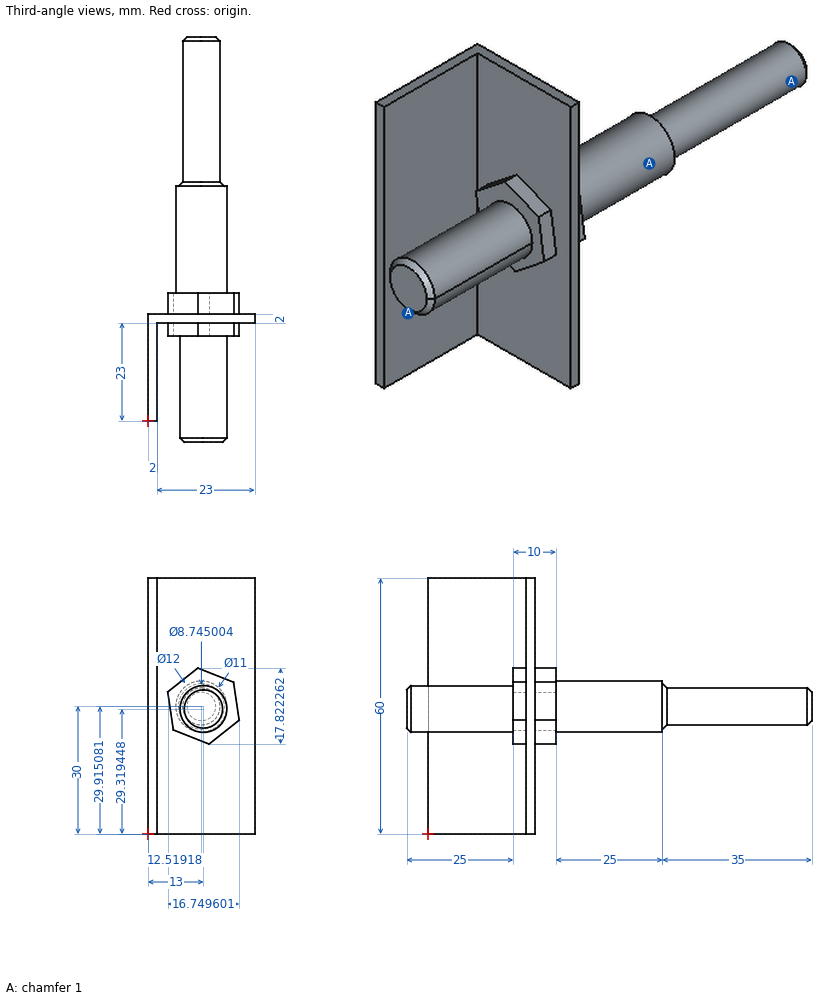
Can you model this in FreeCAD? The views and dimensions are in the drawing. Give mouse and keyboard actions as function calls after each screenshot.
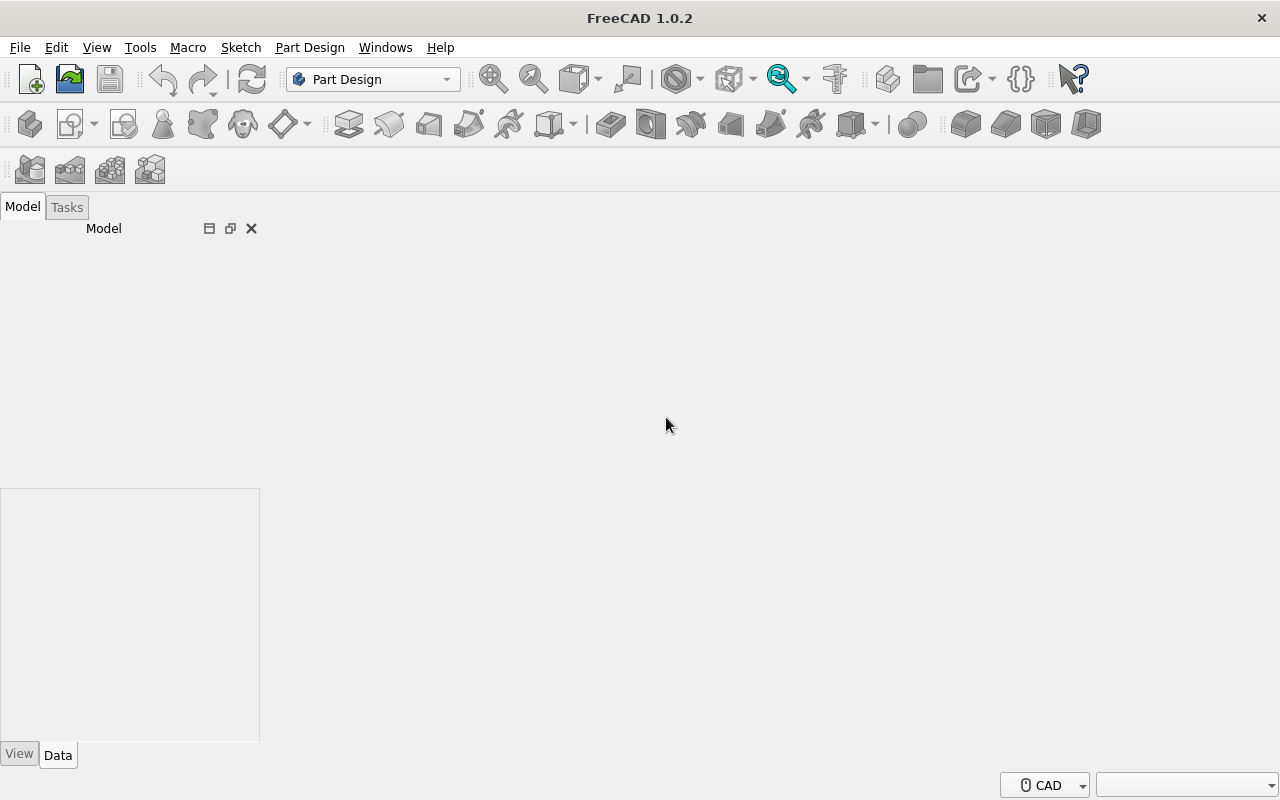
click(30, 80)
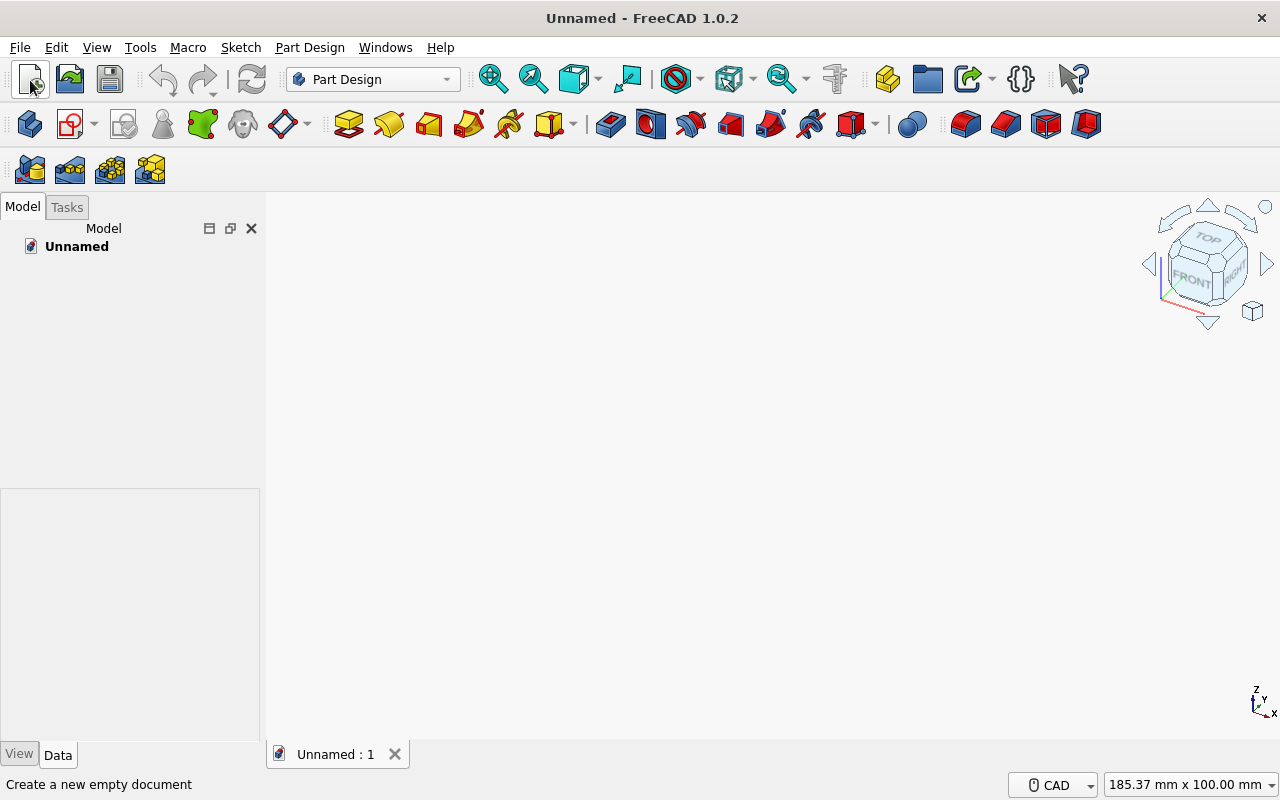
click(70, 124)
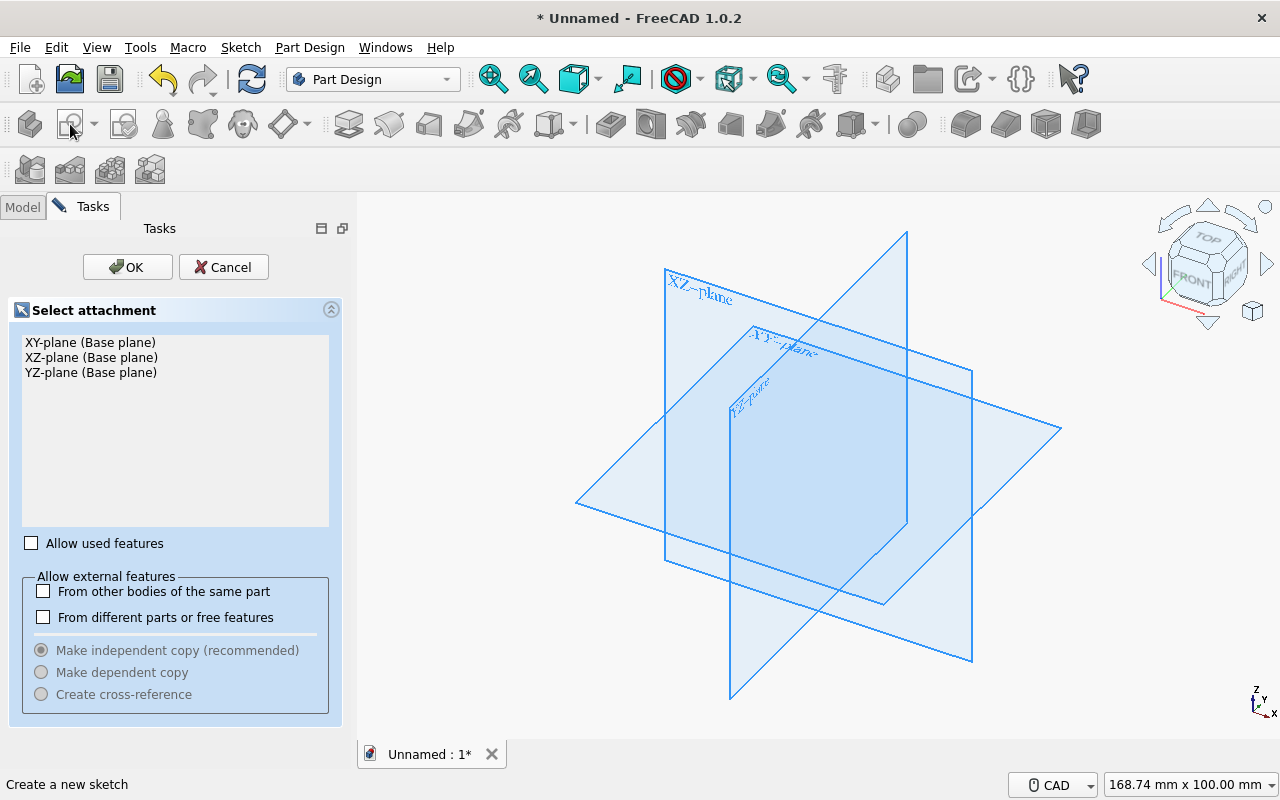
click(82, 342)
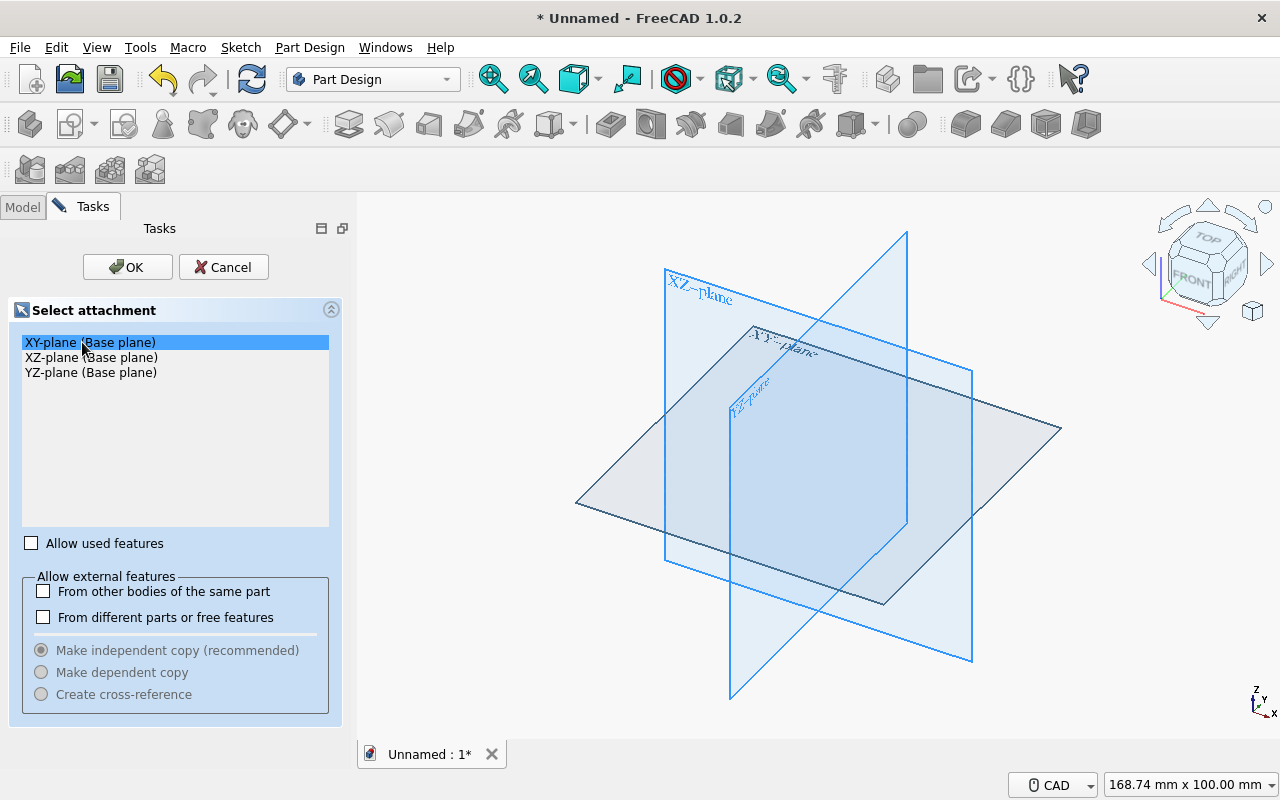
click(128, 267)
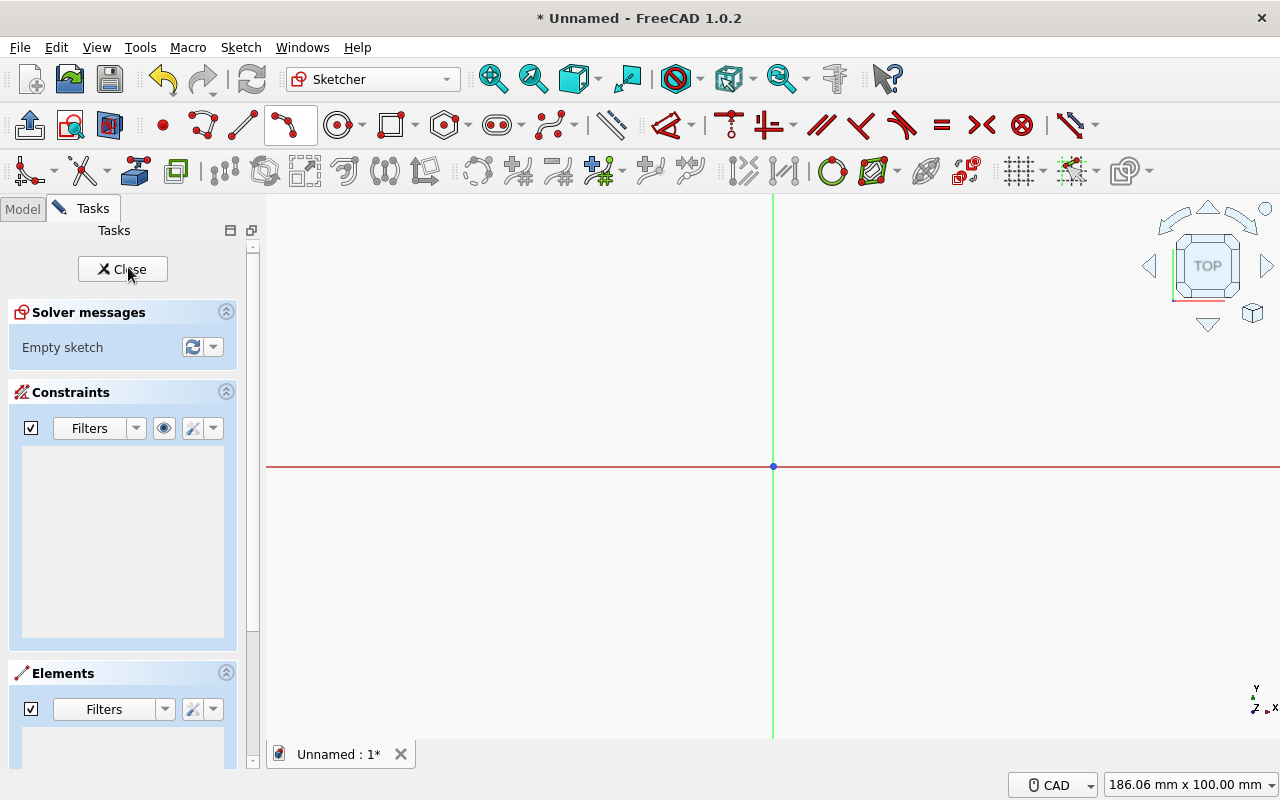
scroll(921, 359, up, 5)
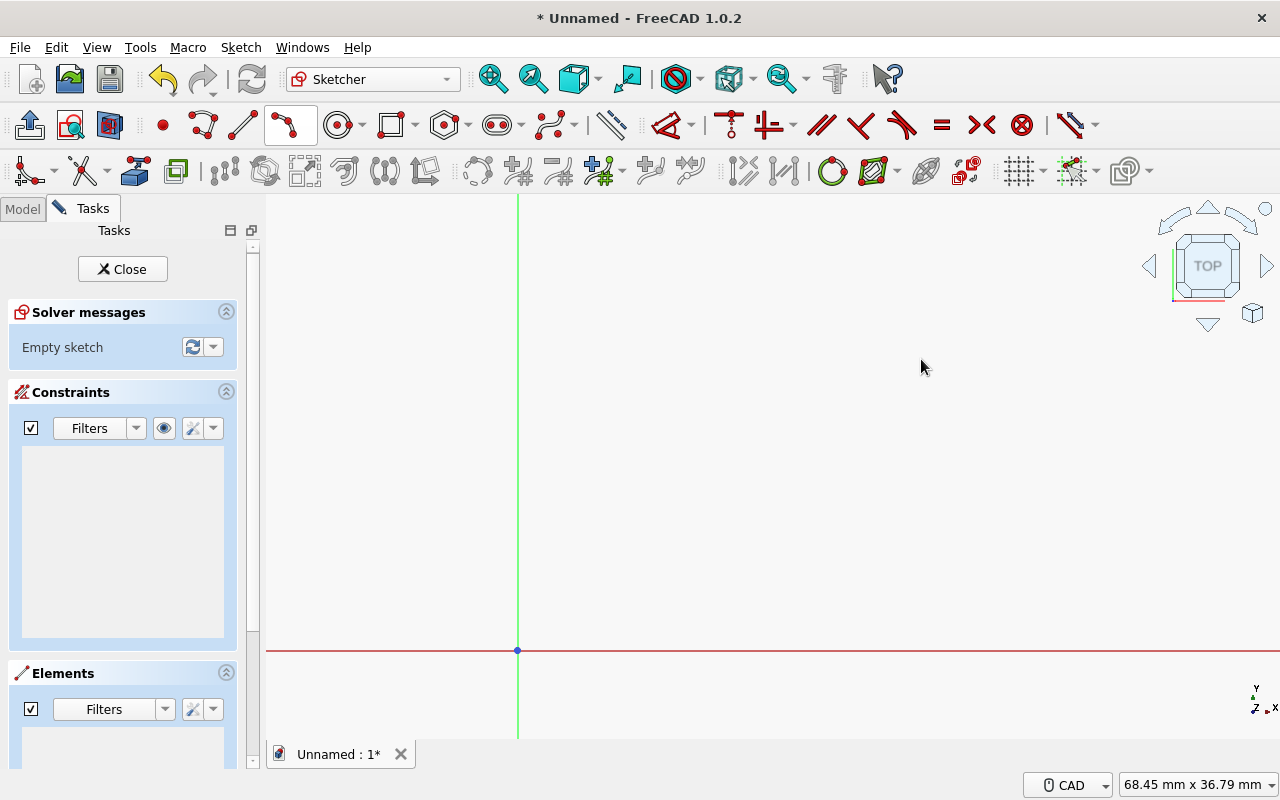
click(204, 126)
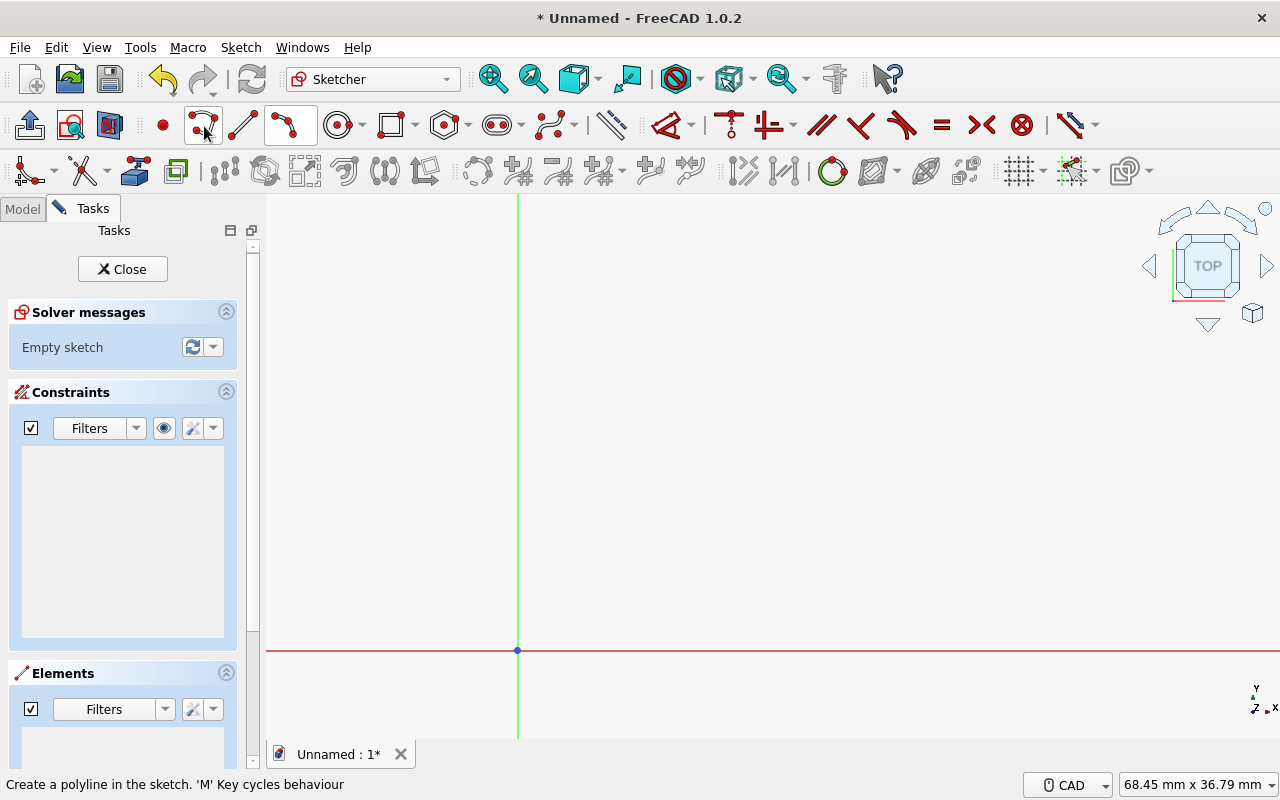
click(518, 651)
click(547, 642)
click(547, 310)
click(888, 310)
click(888, 280)
click(527, 280)
click(518, 651)
key(Escape)
key(Escape)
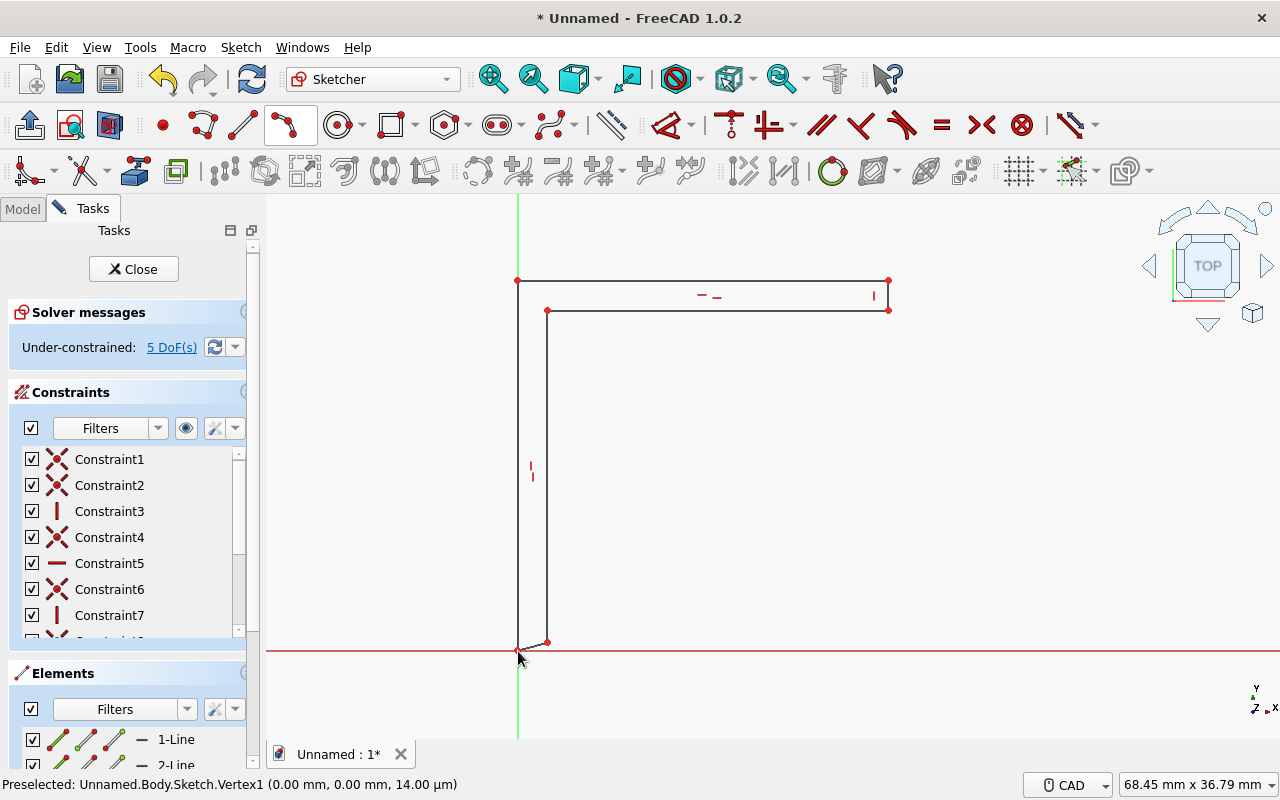
click(529, 648)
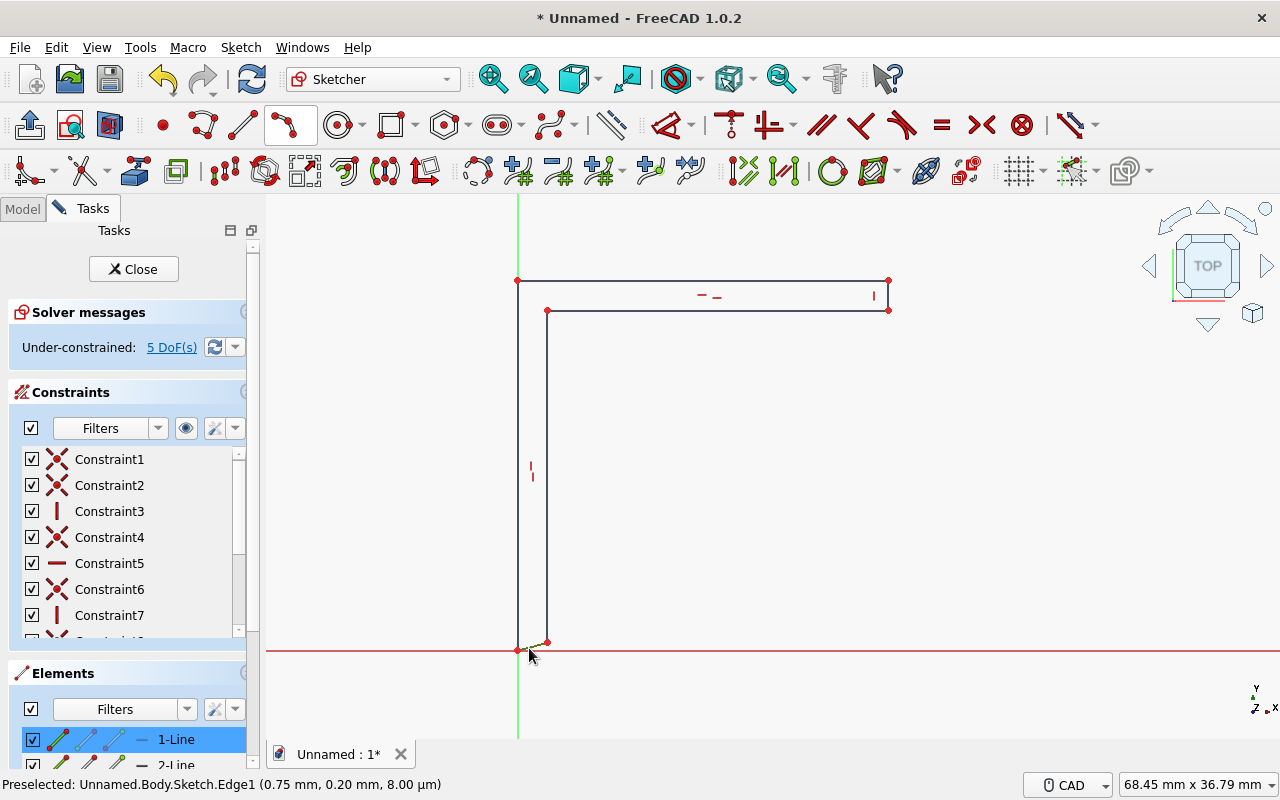
key(h)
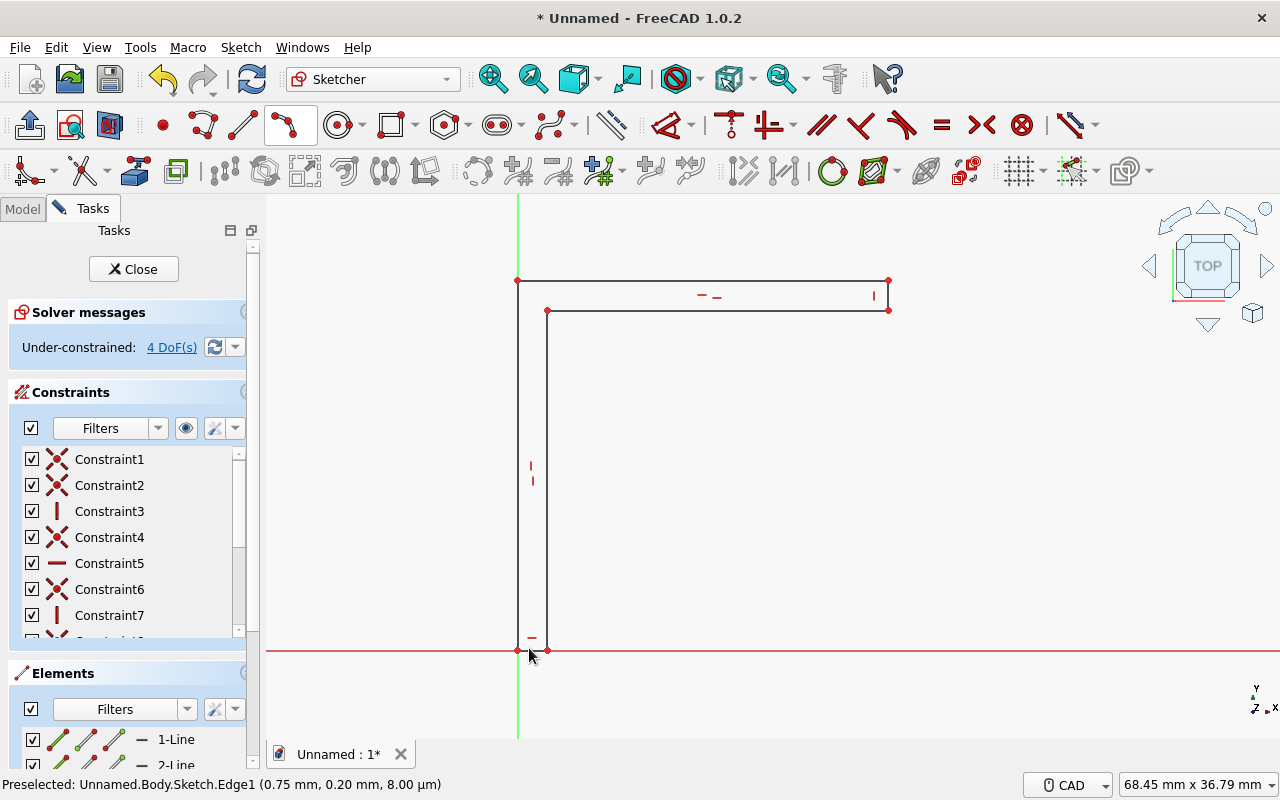
scroll(529, 651, up, 2)